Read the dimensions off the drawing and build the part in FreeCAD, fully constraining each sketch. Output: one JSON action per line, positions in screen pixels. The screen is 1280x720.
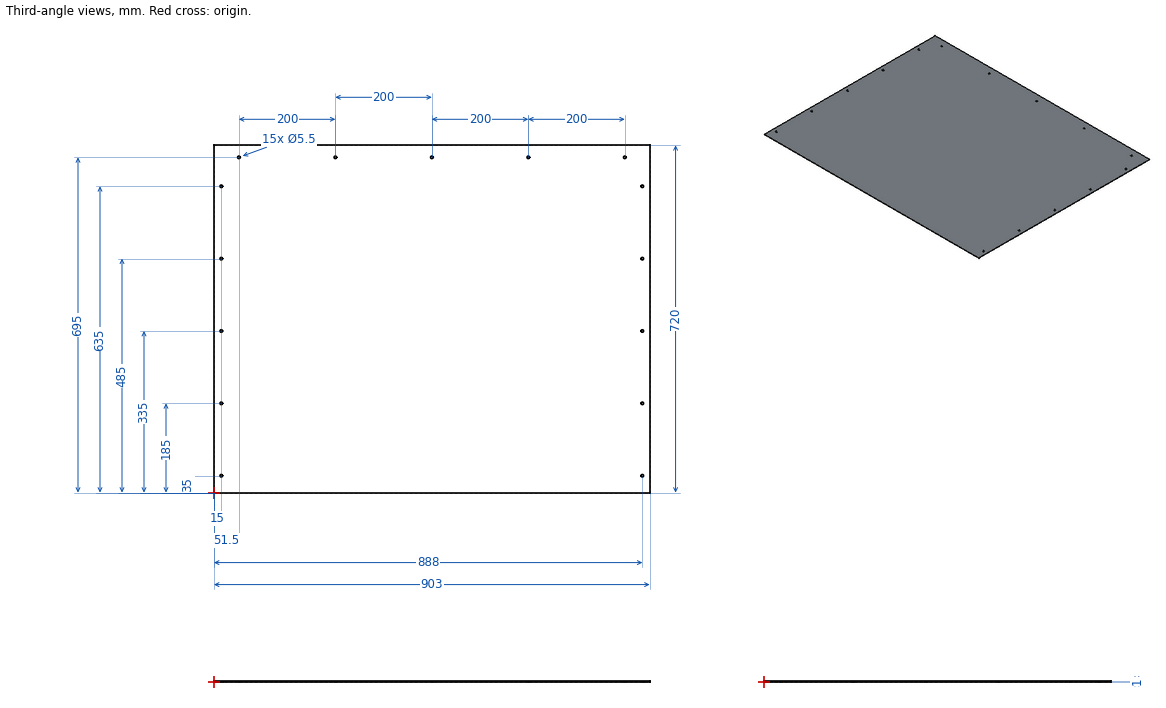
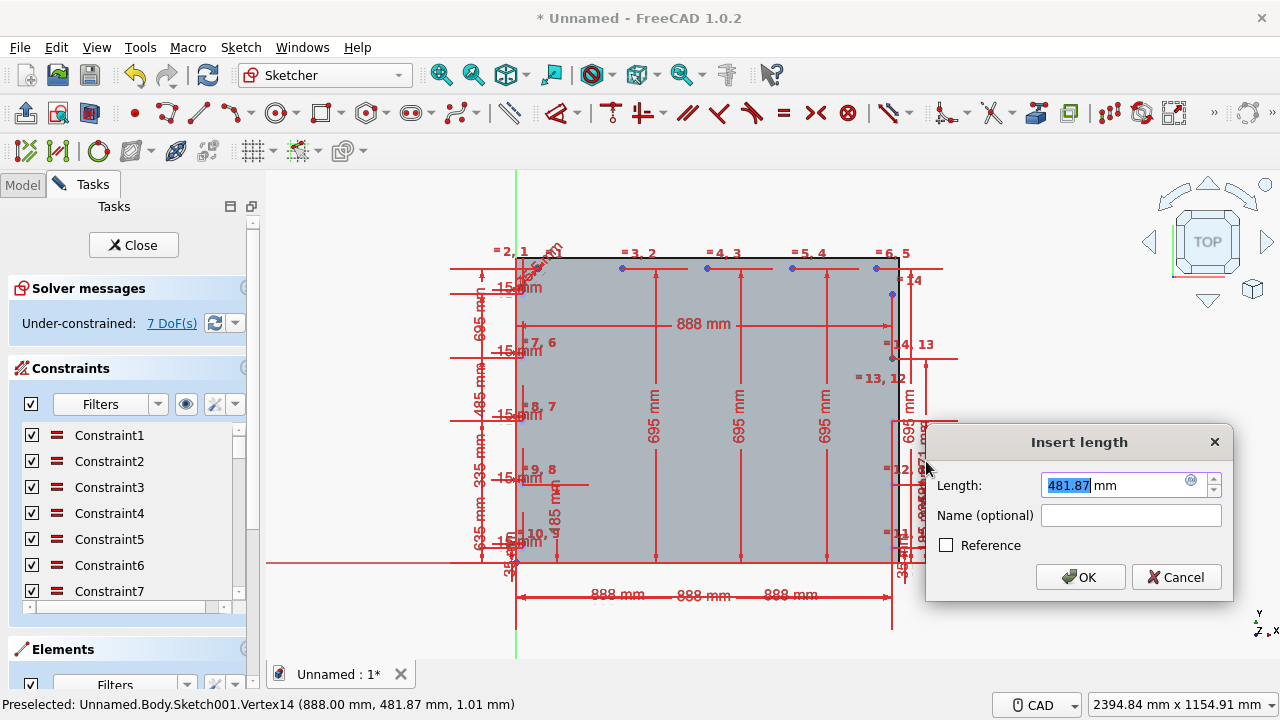
{"action": "type", "text": "485"}
{"action": "key", "text": "Return"}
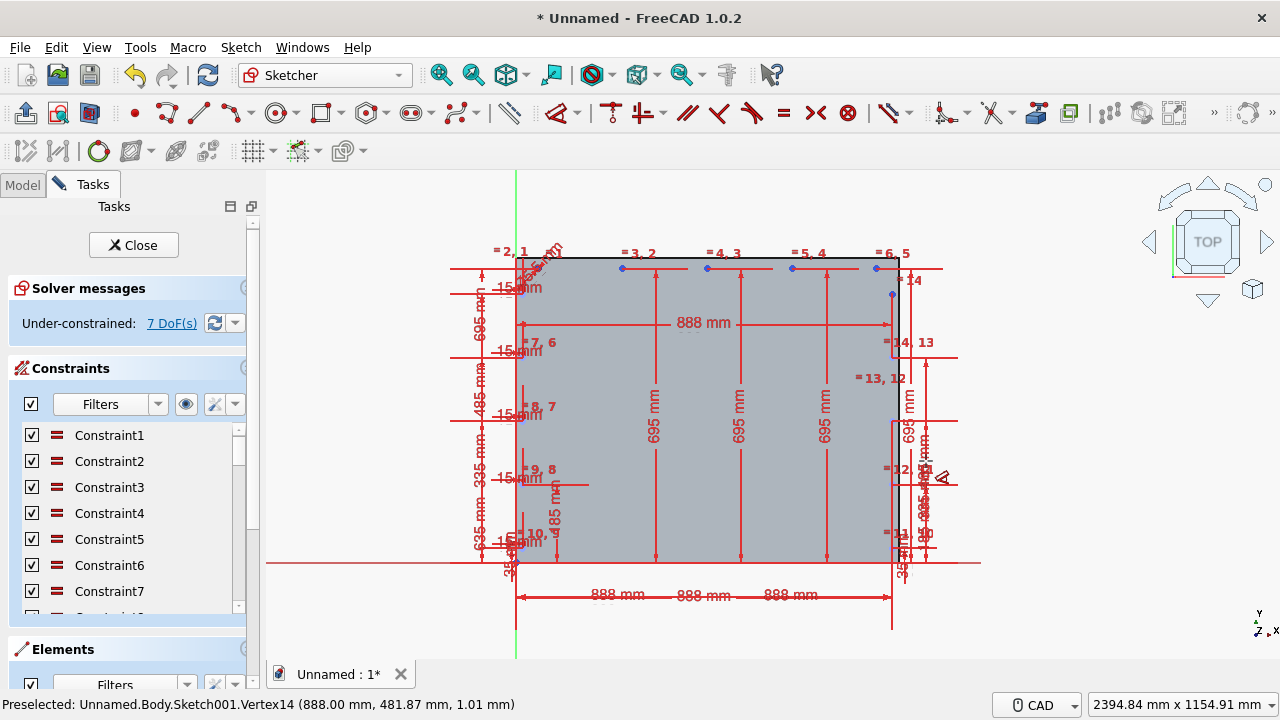
{"action": "left_click", "coordinate": [892, 295]}
{"action": "left_click", "coordinate": [836, 261]}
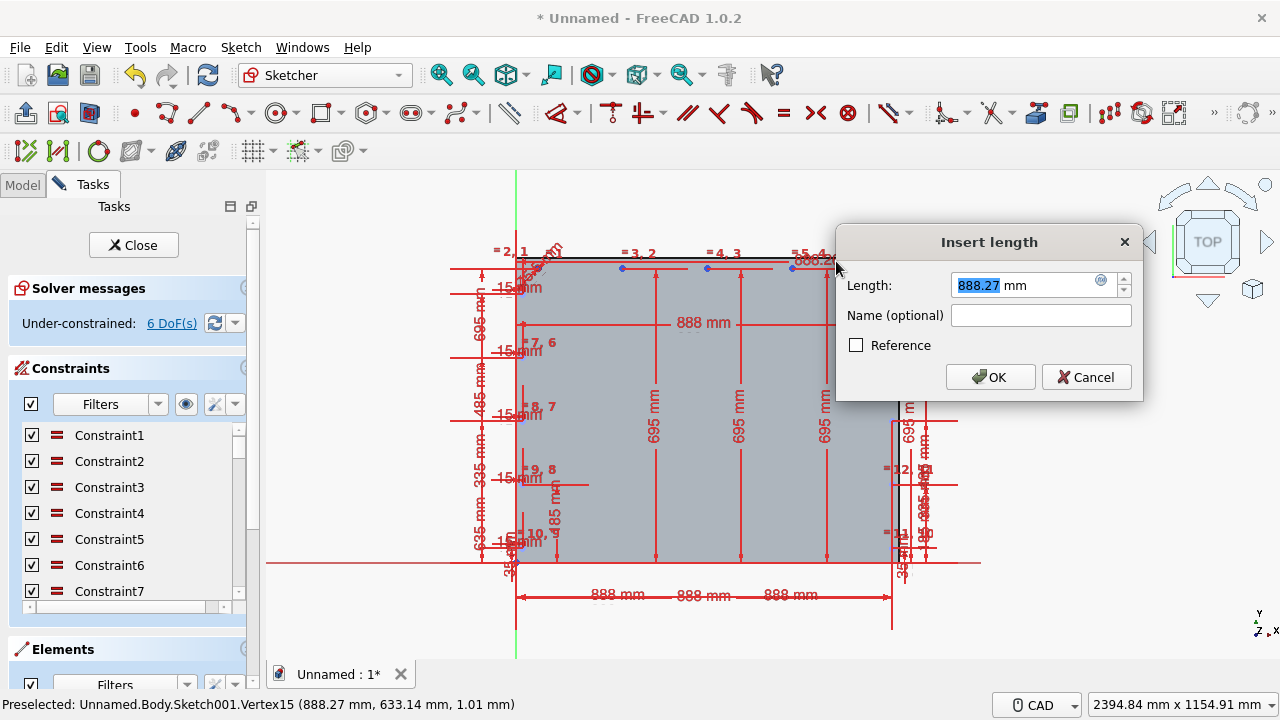
{"action": "type", "text": "888"}
{"action": "key", "text": "Return"}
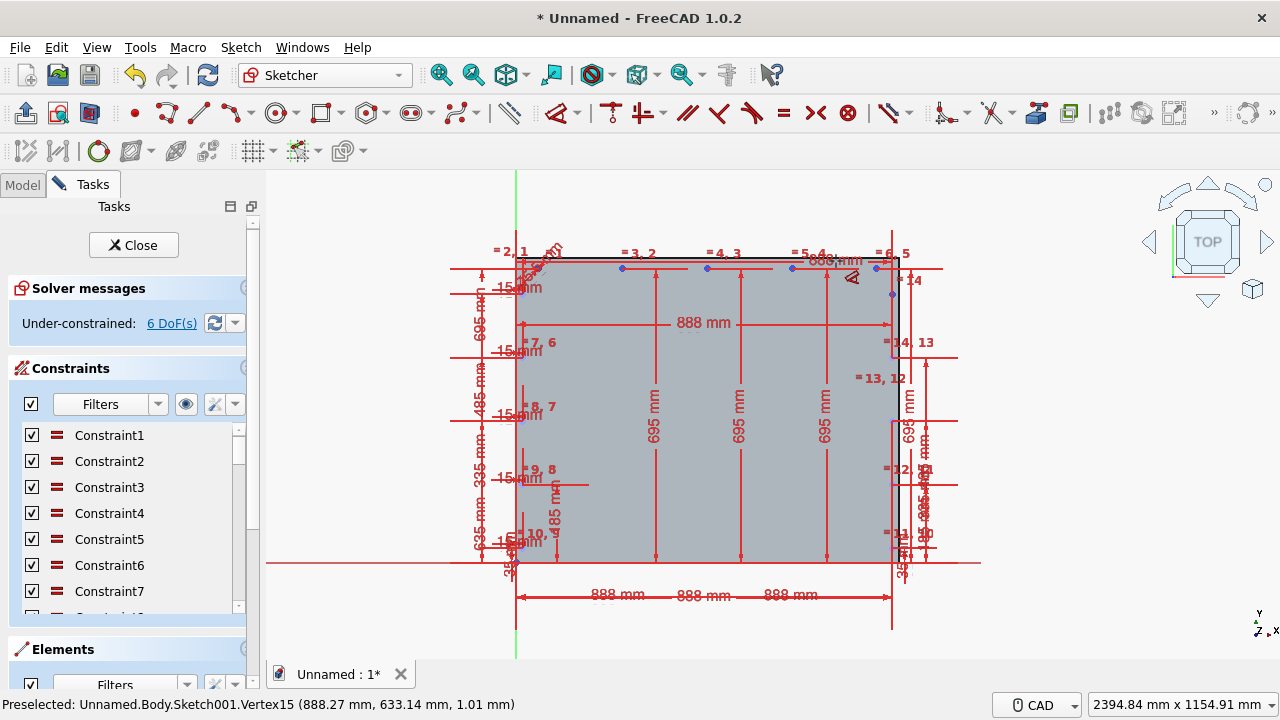
{"action": "left_click", "coordinate": [892, 295]}
{"action": "left_click", "coordinate": [926, 367]}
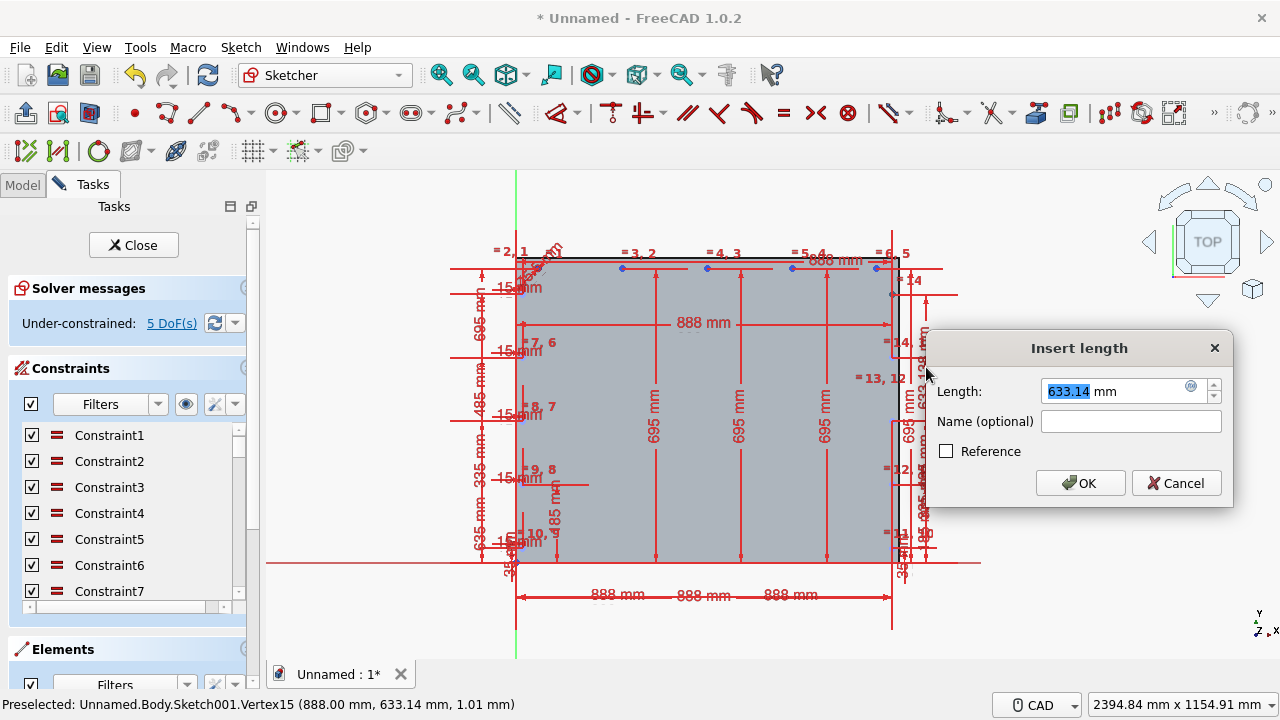
{"action": "type", "text": "635"}
{"action": "key", "text": "Return"}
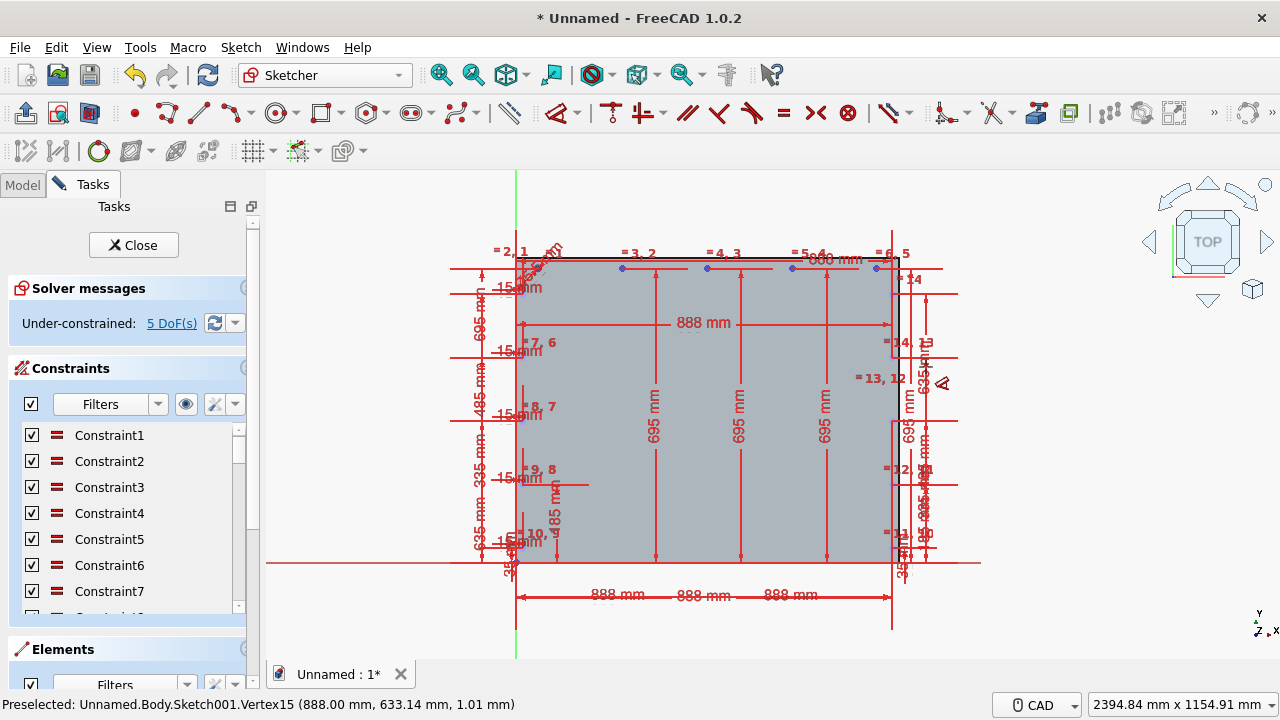
{"action": "scroll", "coordinate": [538, 269], "scroll_direction": "up", "scroll_amount": 3}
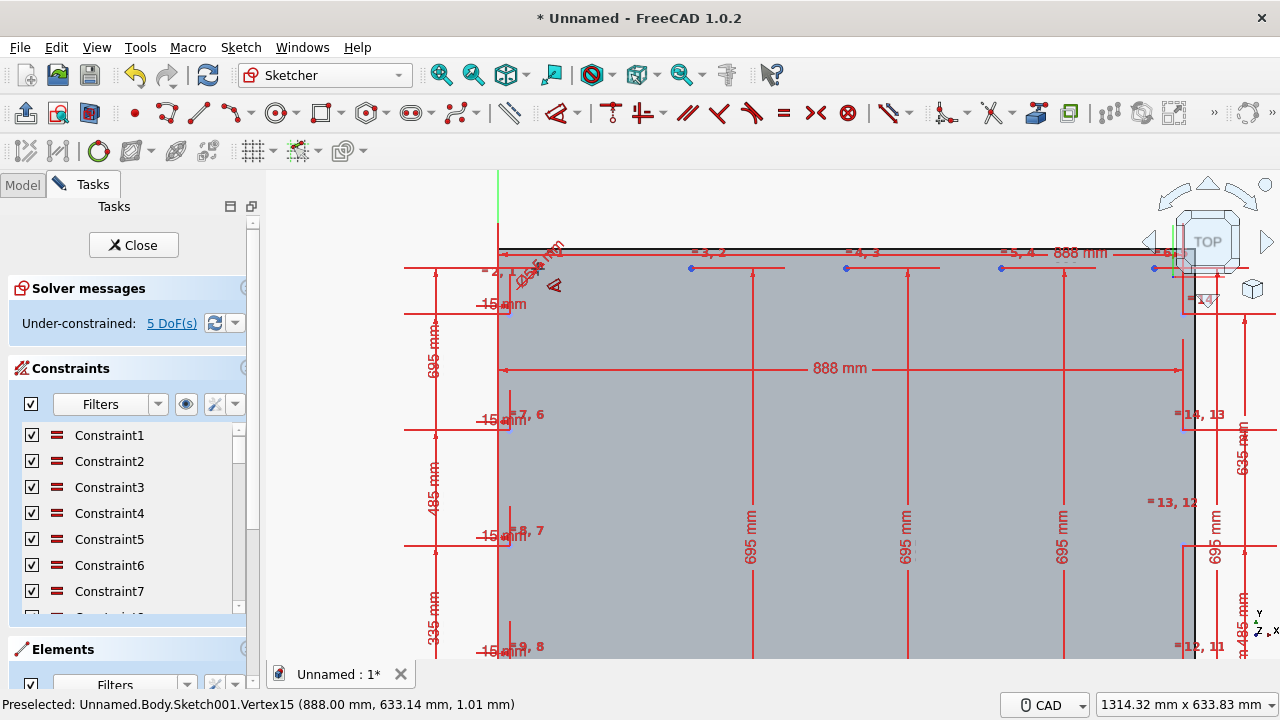
{"action": "left_click", "coordinate": [538, 268]}
{"action": "left_click", "coordinate": [518, 234]}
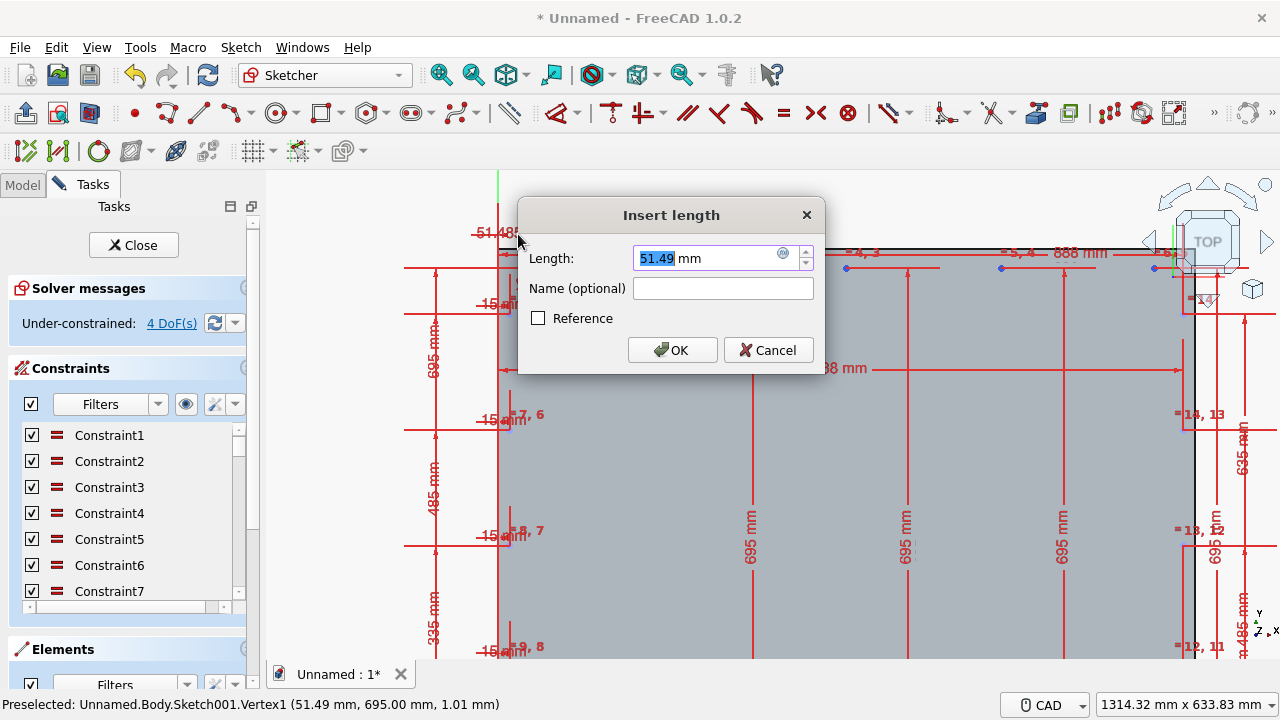
{"action": "type", "text": "51.5"}
{"action": "key", "text": "Return"}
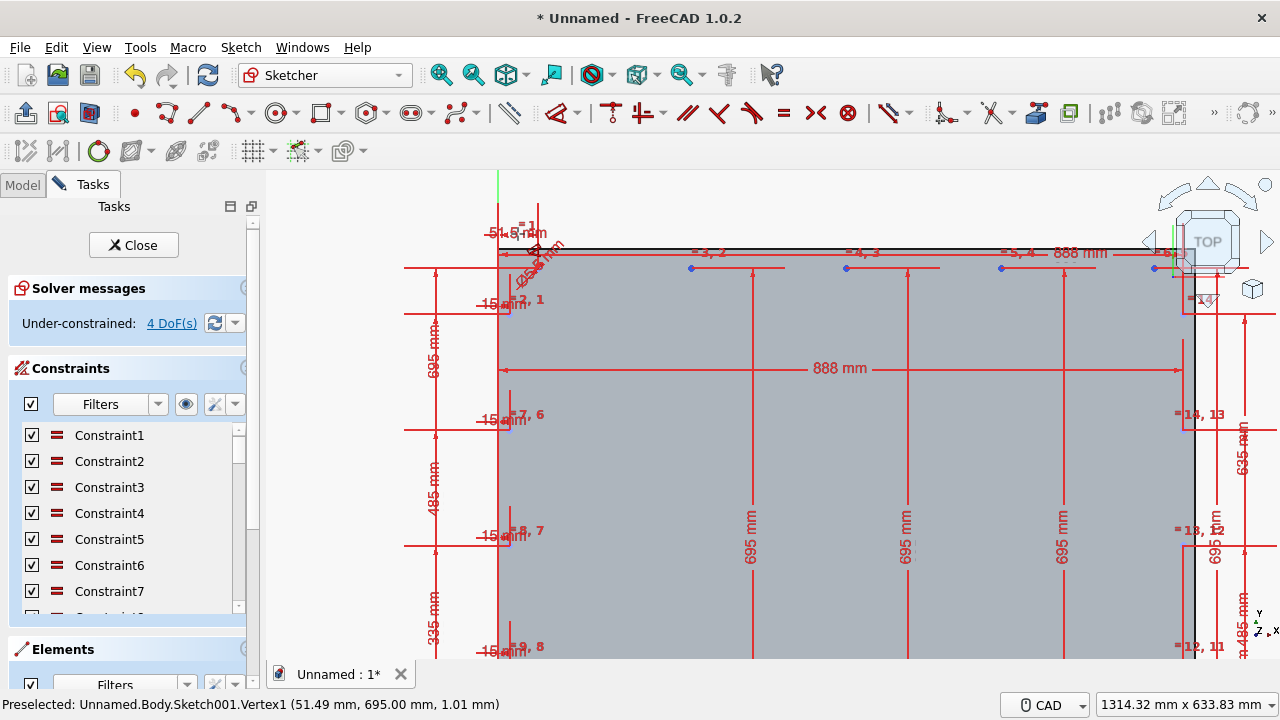
{"action": "left_click", "coordinate": [538, 268]}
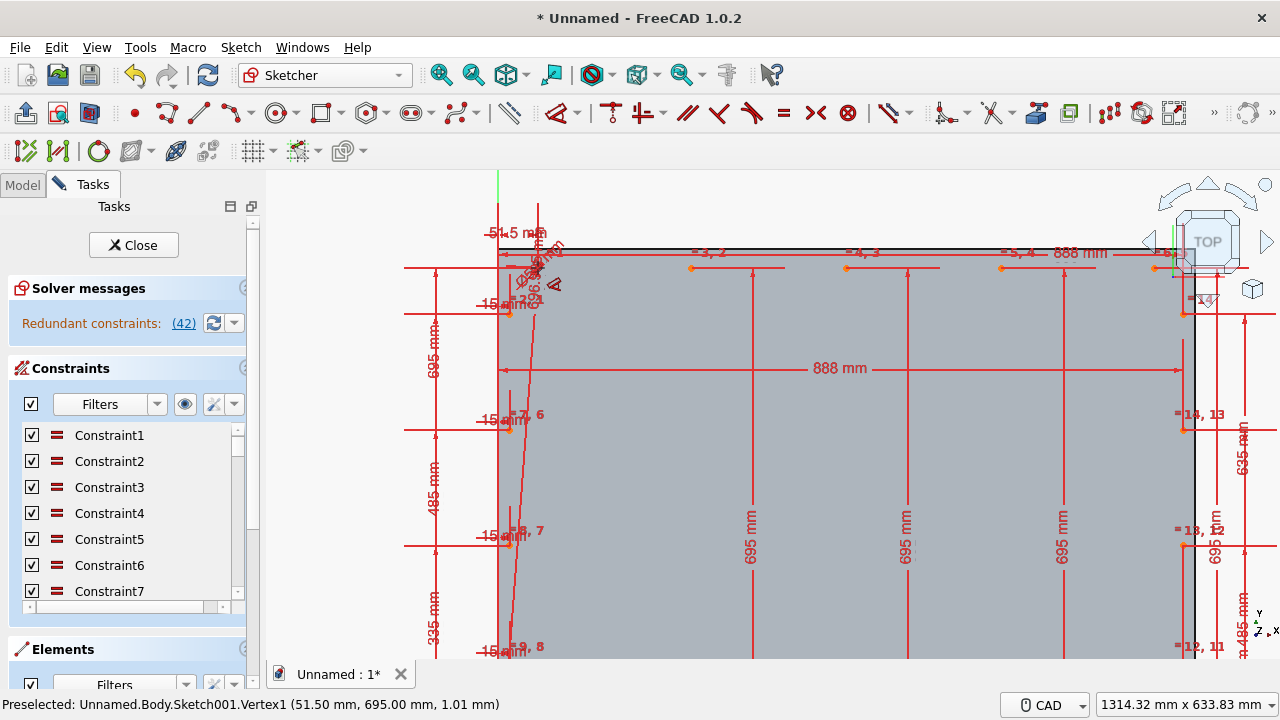
{"action": "left_click", "coordinate": [692, 268]}
{"action": "left_click", "coordinate": [615, 234]}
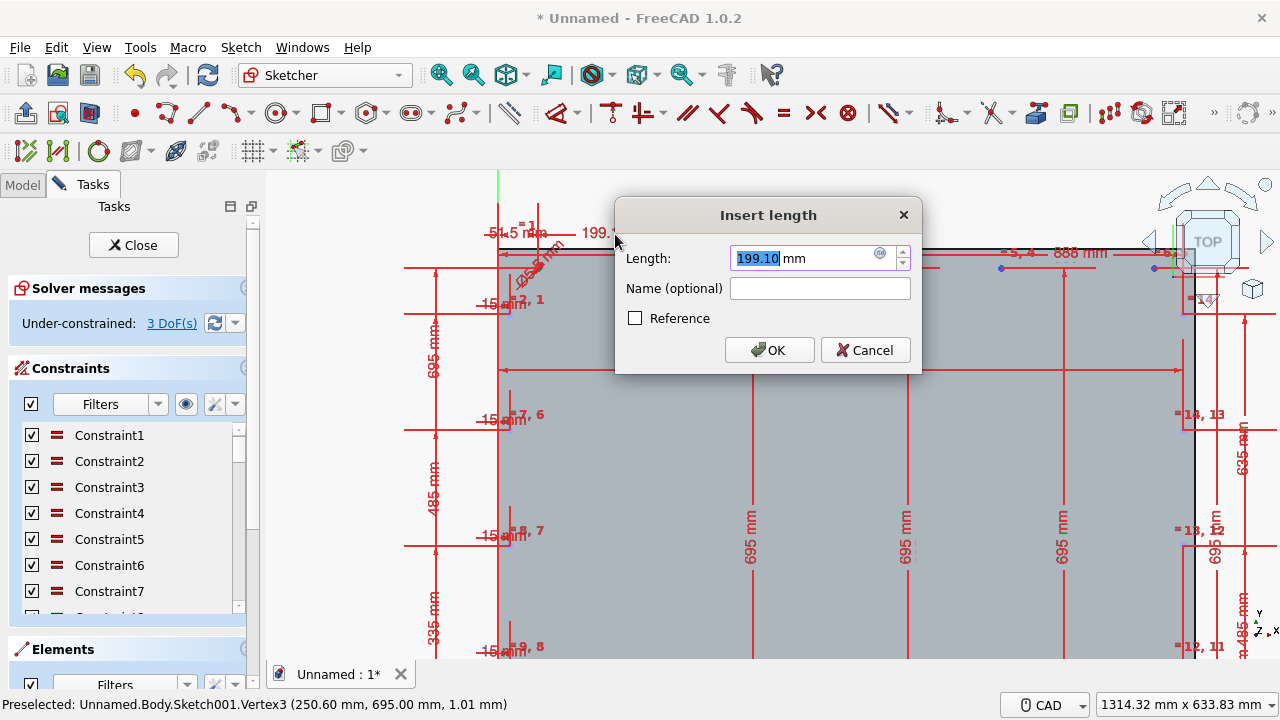
{"action": "type", "text": "200"}
{"action": "key", "text": "Return"}